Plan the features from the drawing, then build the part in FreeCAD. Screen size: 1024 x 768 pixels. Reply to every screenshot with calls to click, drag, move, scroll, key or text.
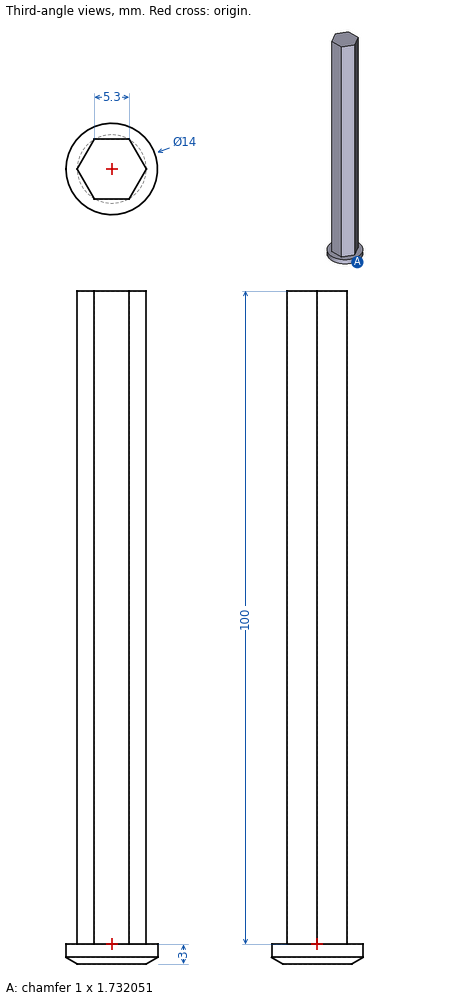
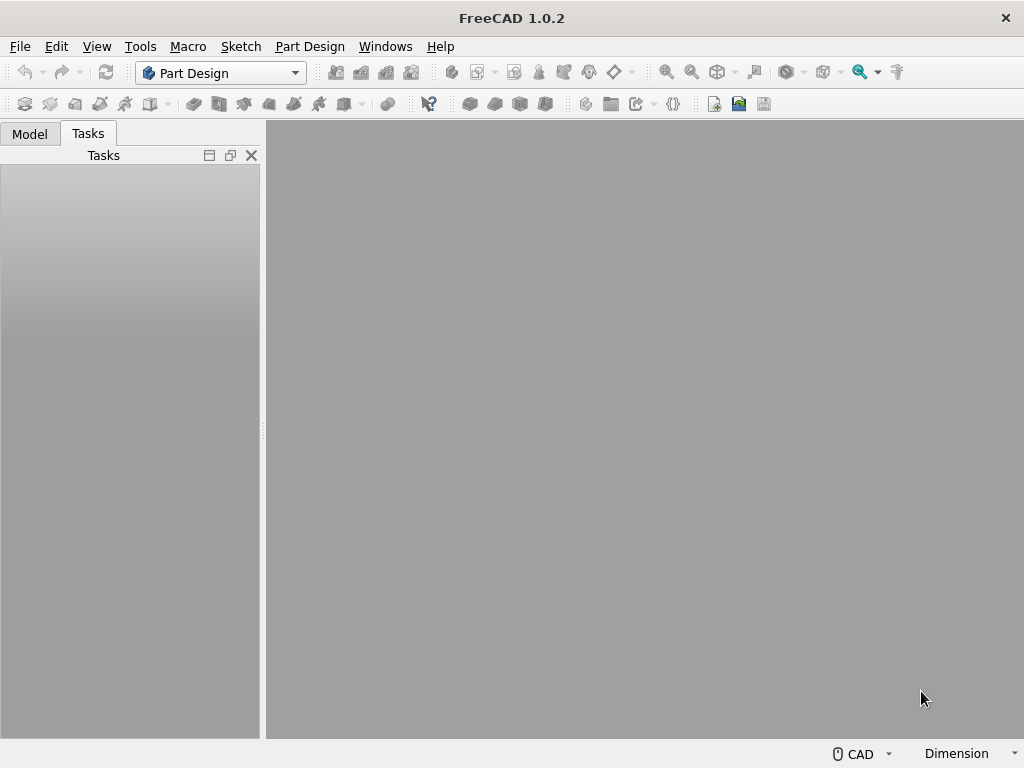
click(714, 104)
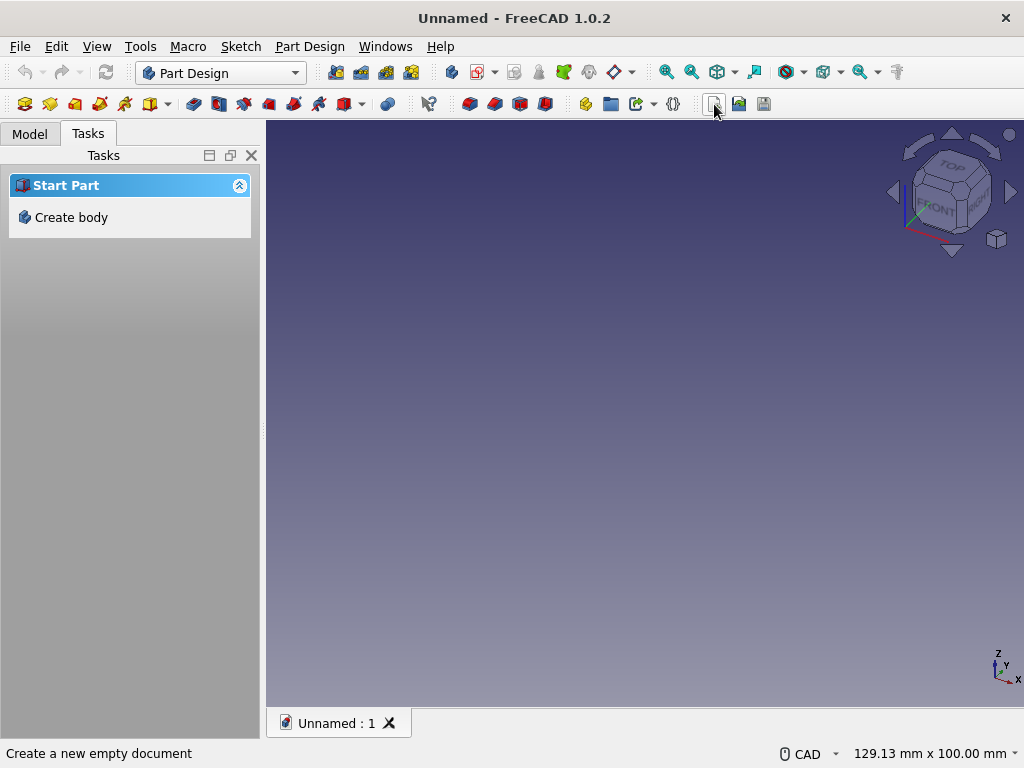
click(476, 72)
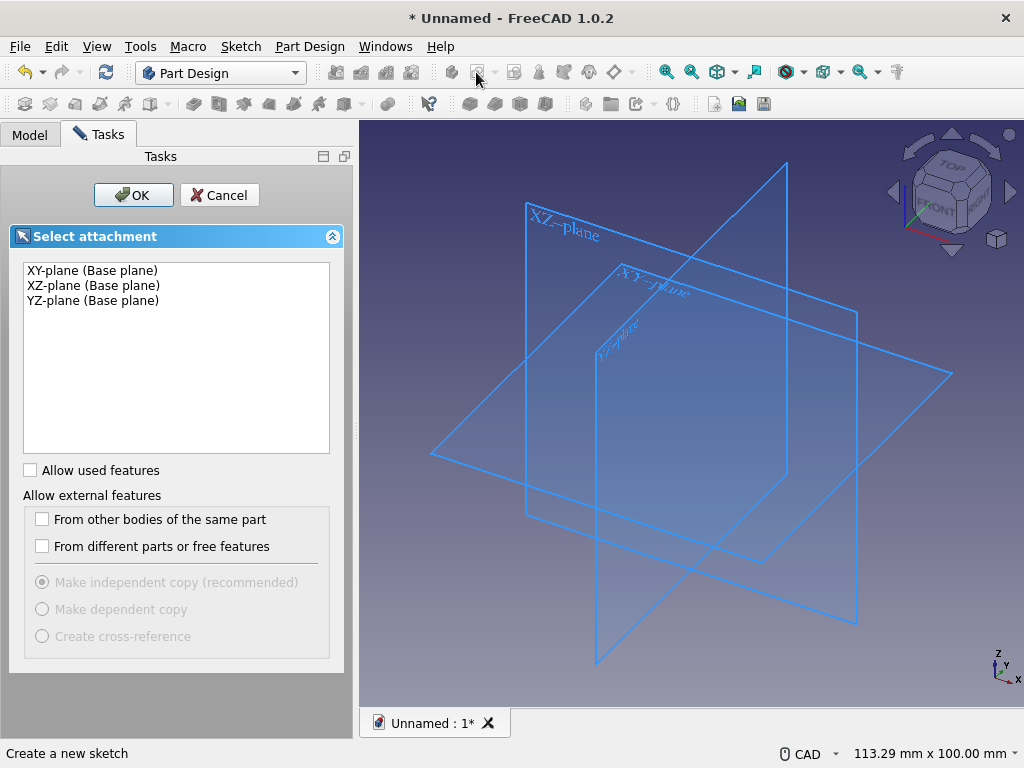
click(84, 270)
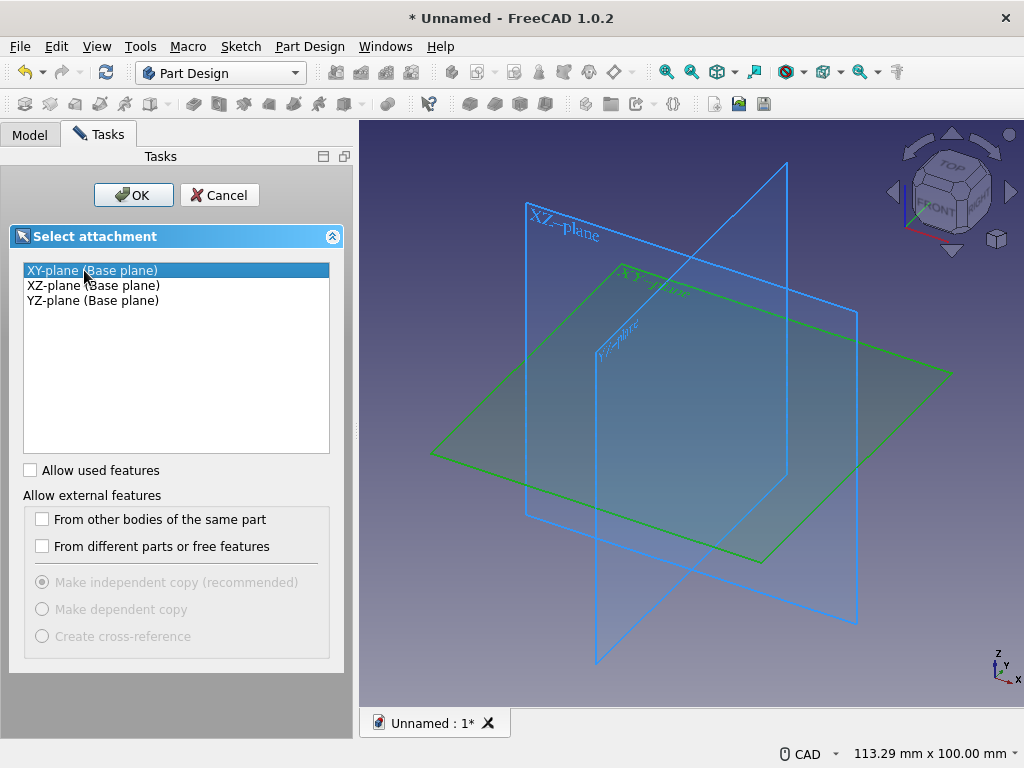
click(134, 195)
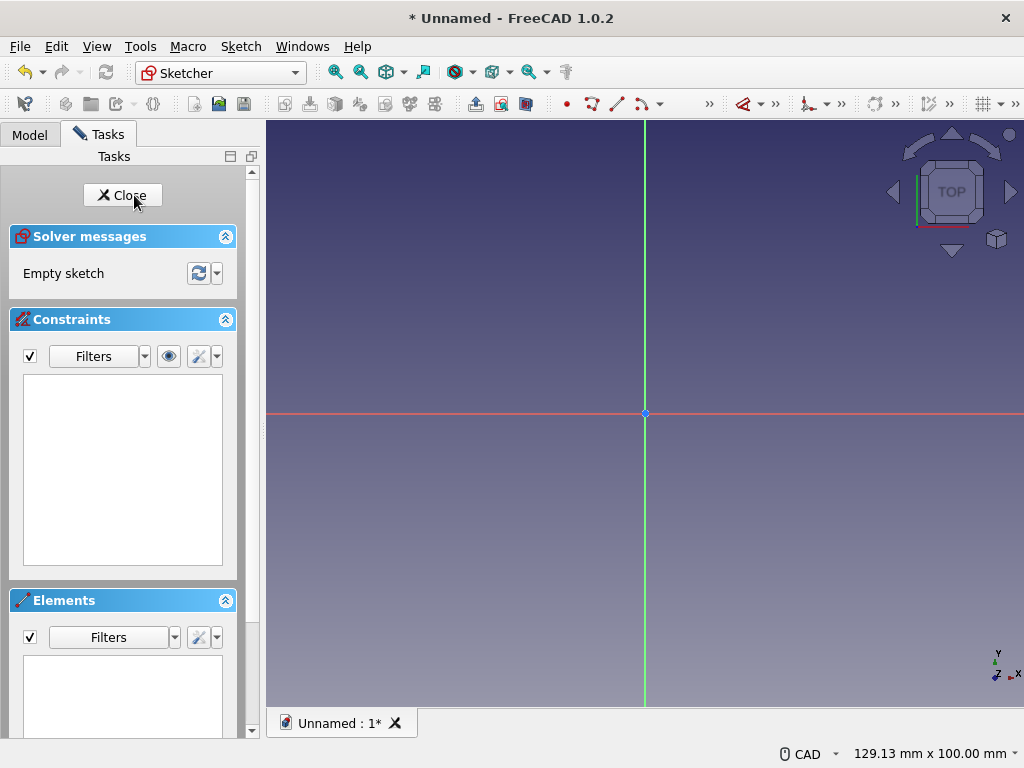
scroll(659, 414, up, 9)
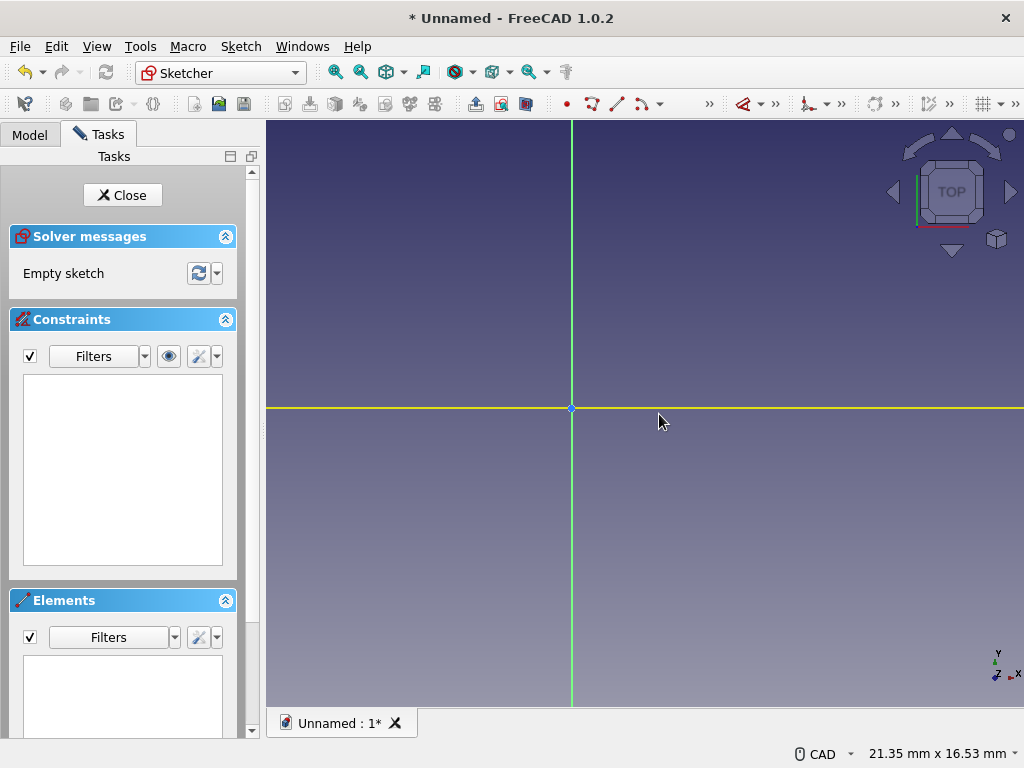
key(g)
key(p)
key(6)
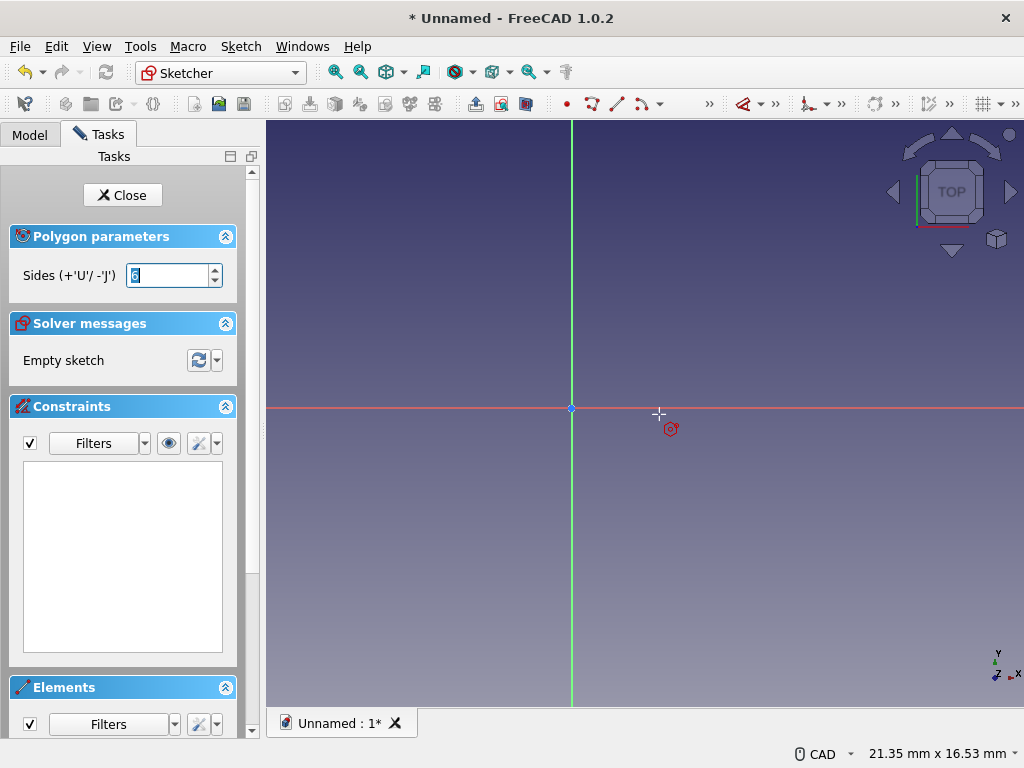
click(572, 408)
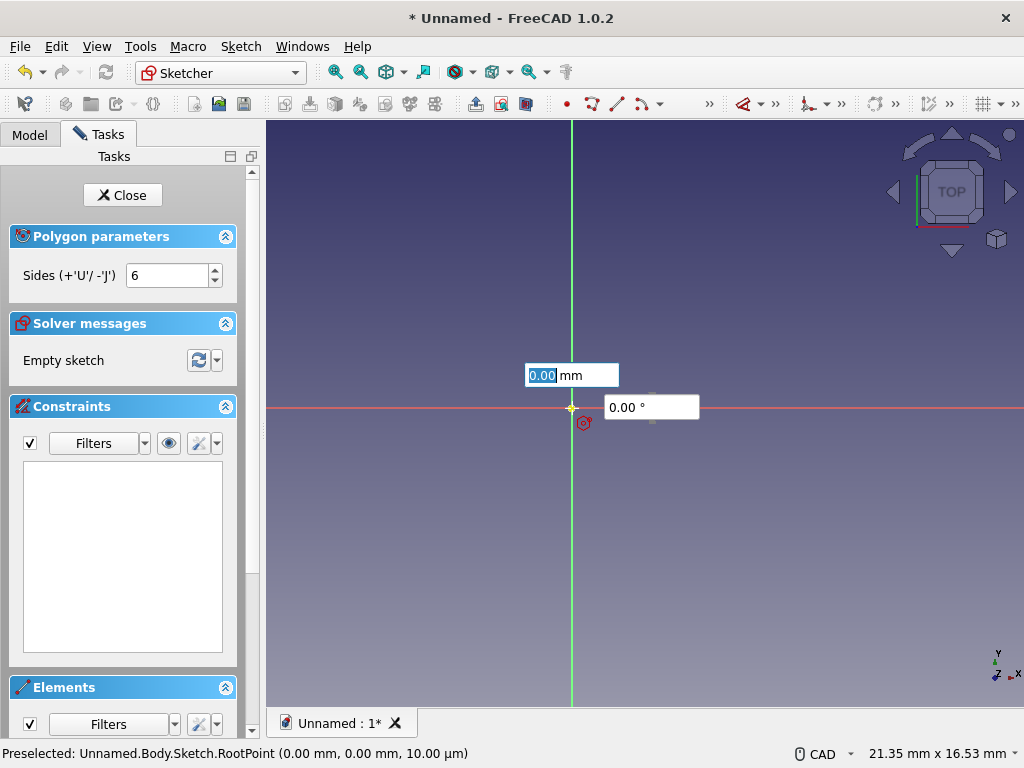
click(760, 408)
right_click(760, 408)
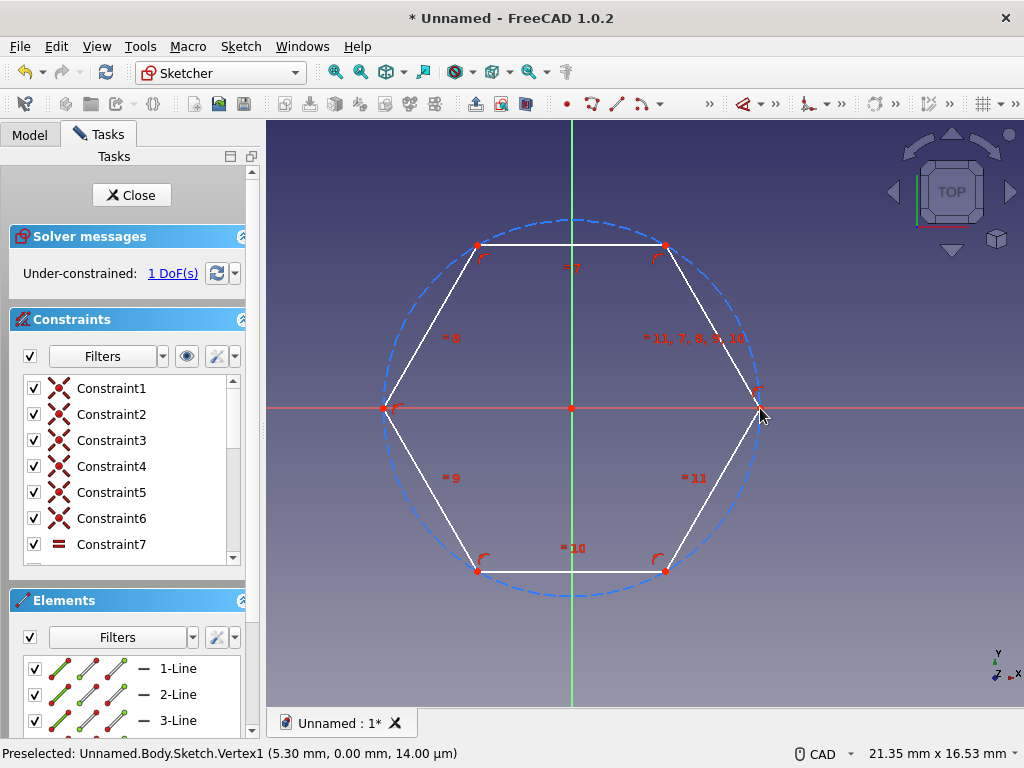
click(609, 245)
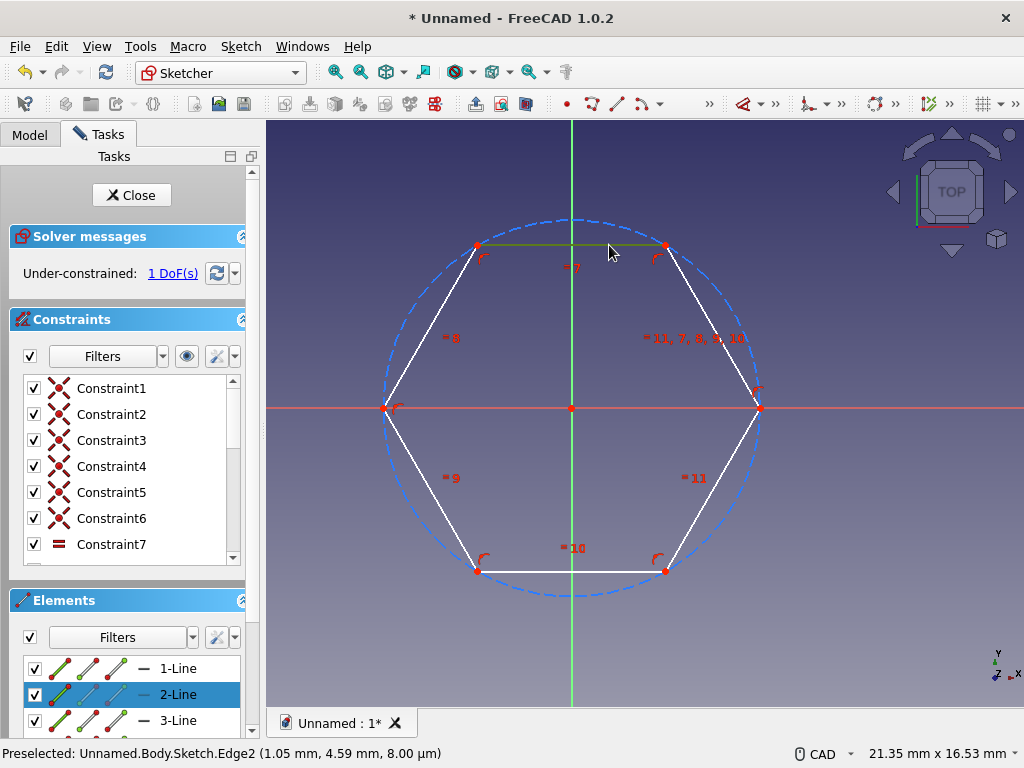
click(760, 104)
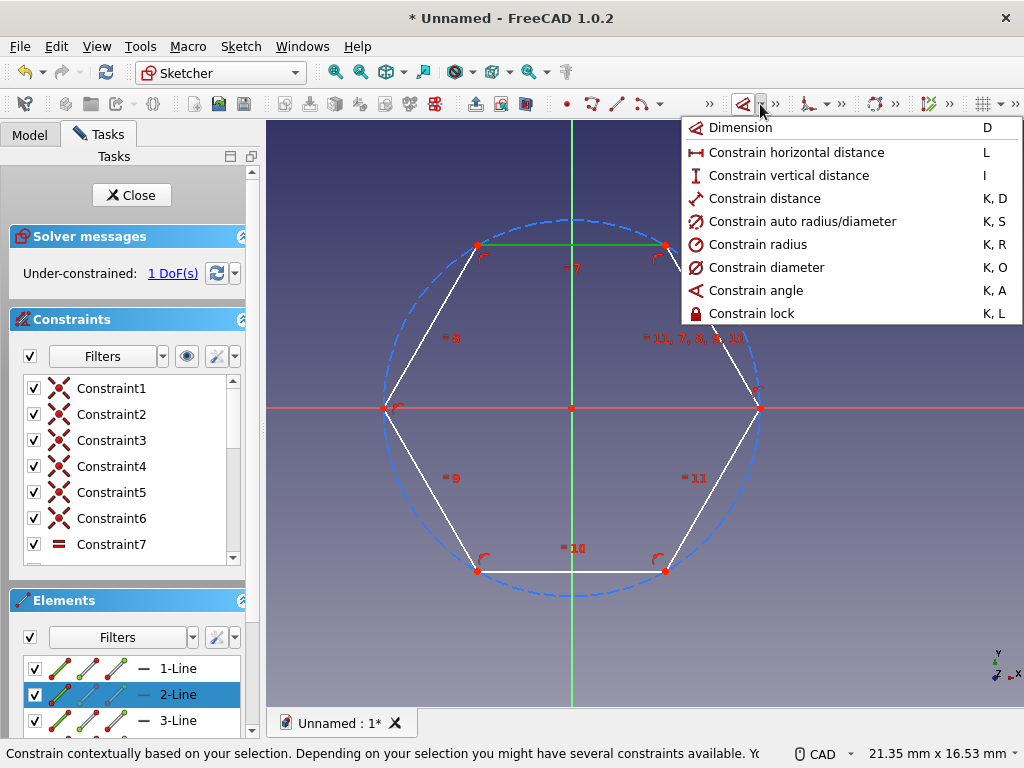
click(852, 152)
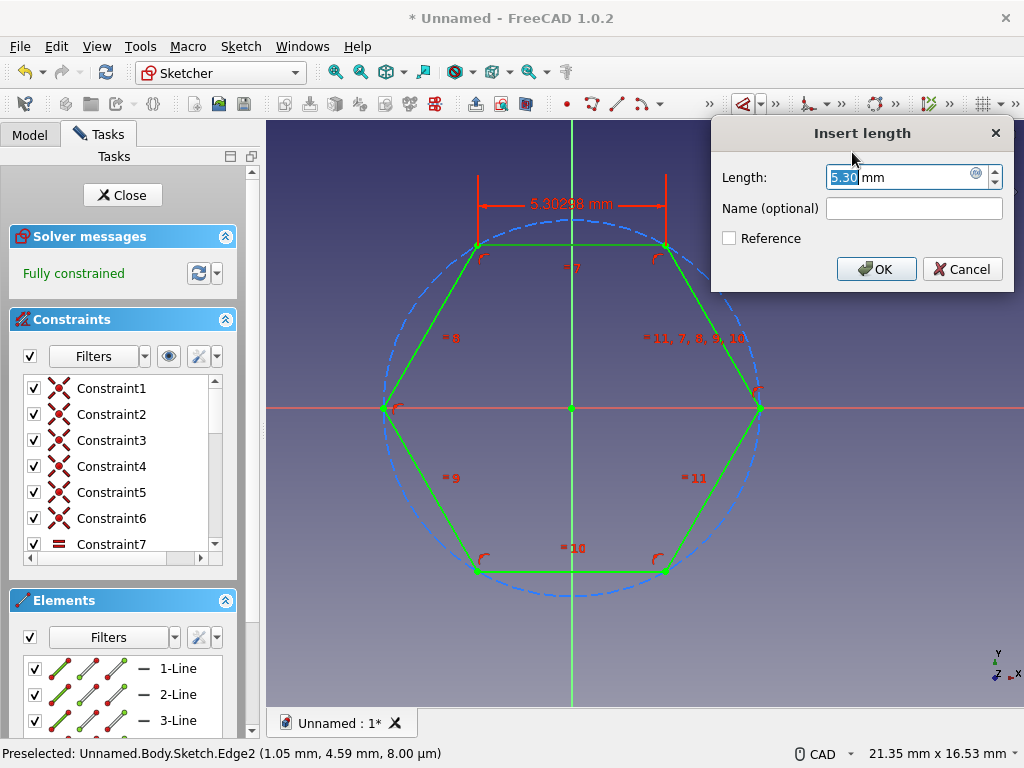
text(5.3)
key(Return)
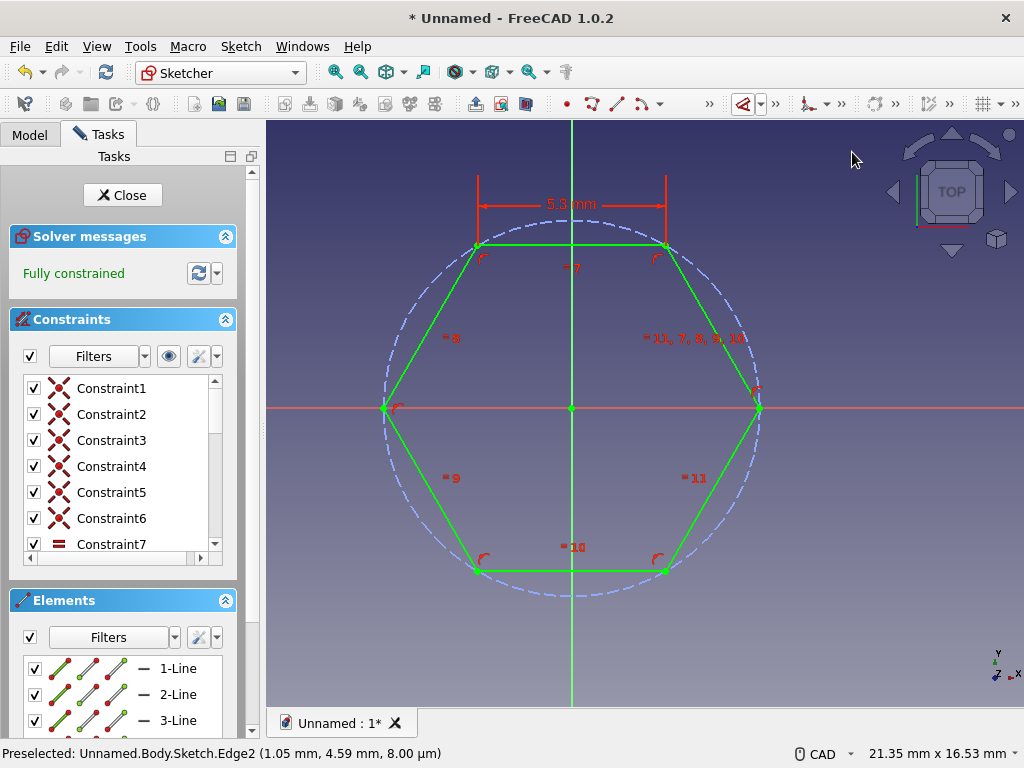
click(123, 195)